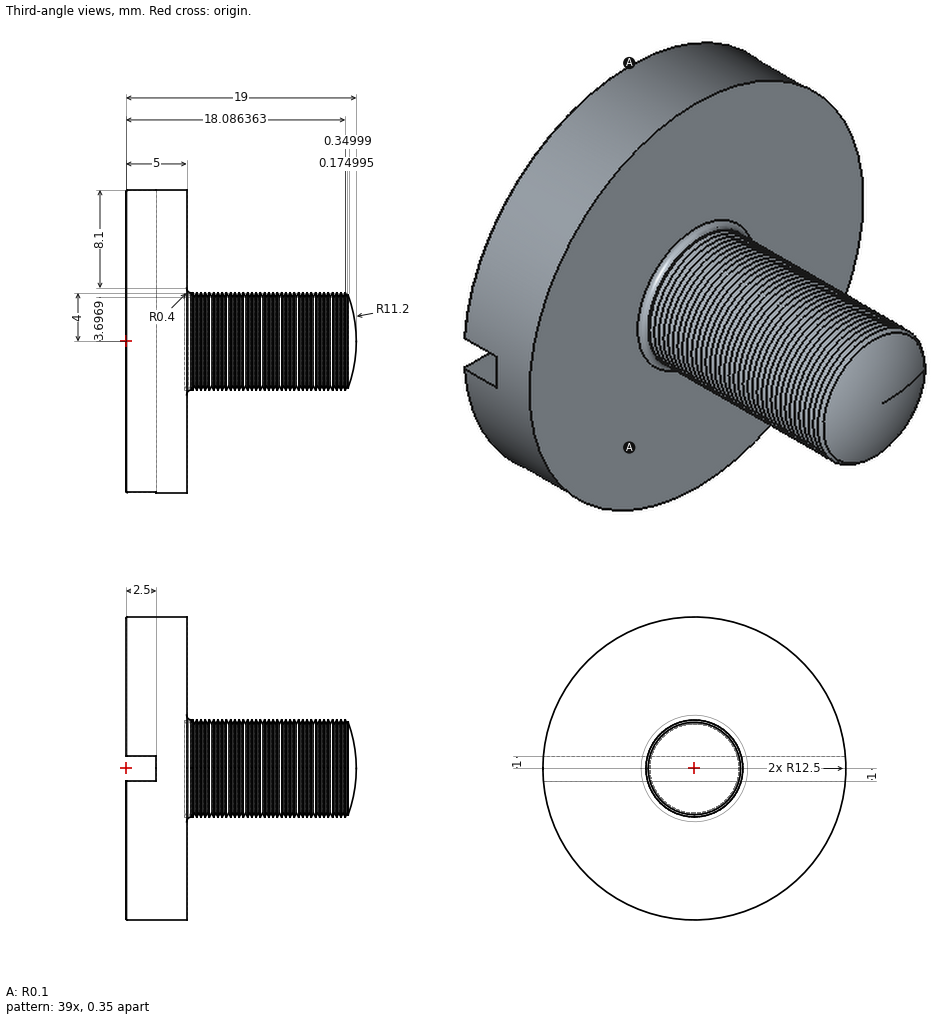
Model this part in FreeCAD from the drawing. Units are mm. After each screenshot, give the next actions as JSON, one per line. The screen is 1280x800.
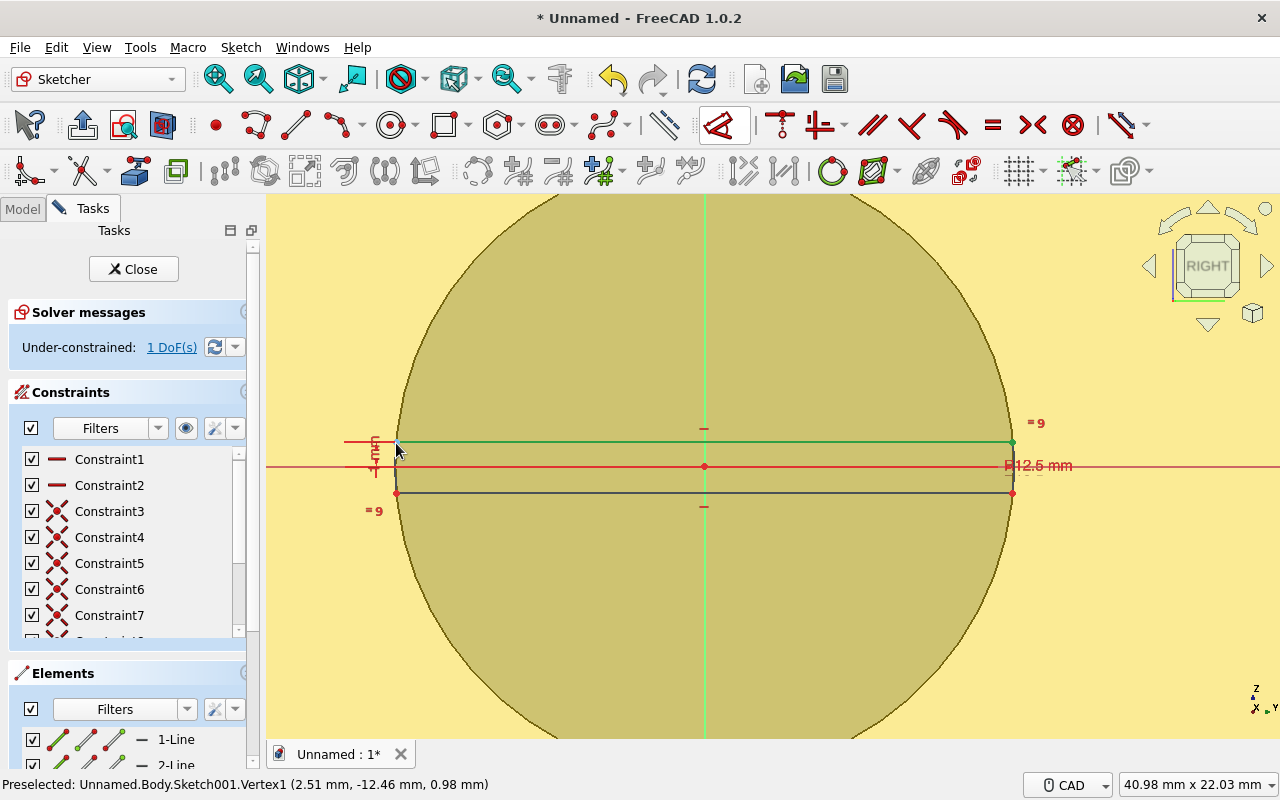
{"action": "scroll", "coordinate": [1013, 493], "scroll_direction": "up", "scroll_amount": 3}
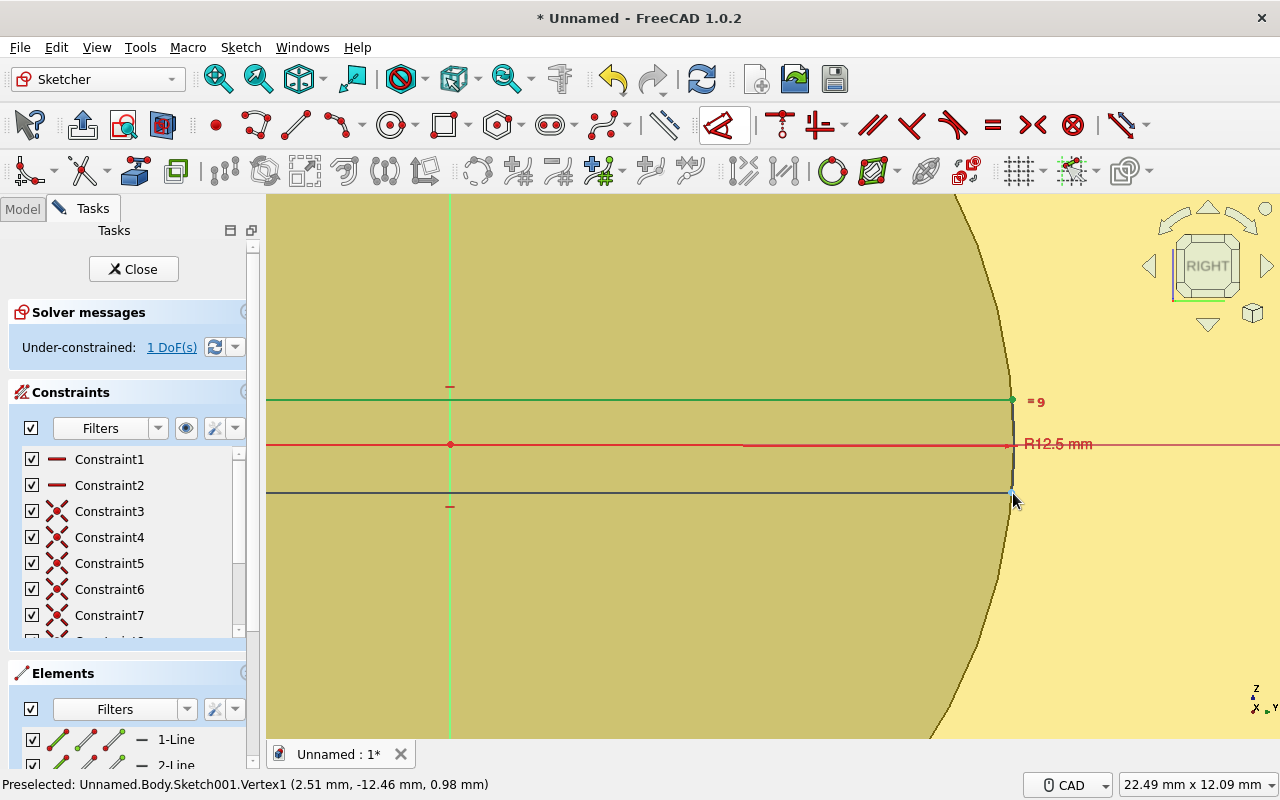
{"action": "left_click", "coordinate": [1012, 493]}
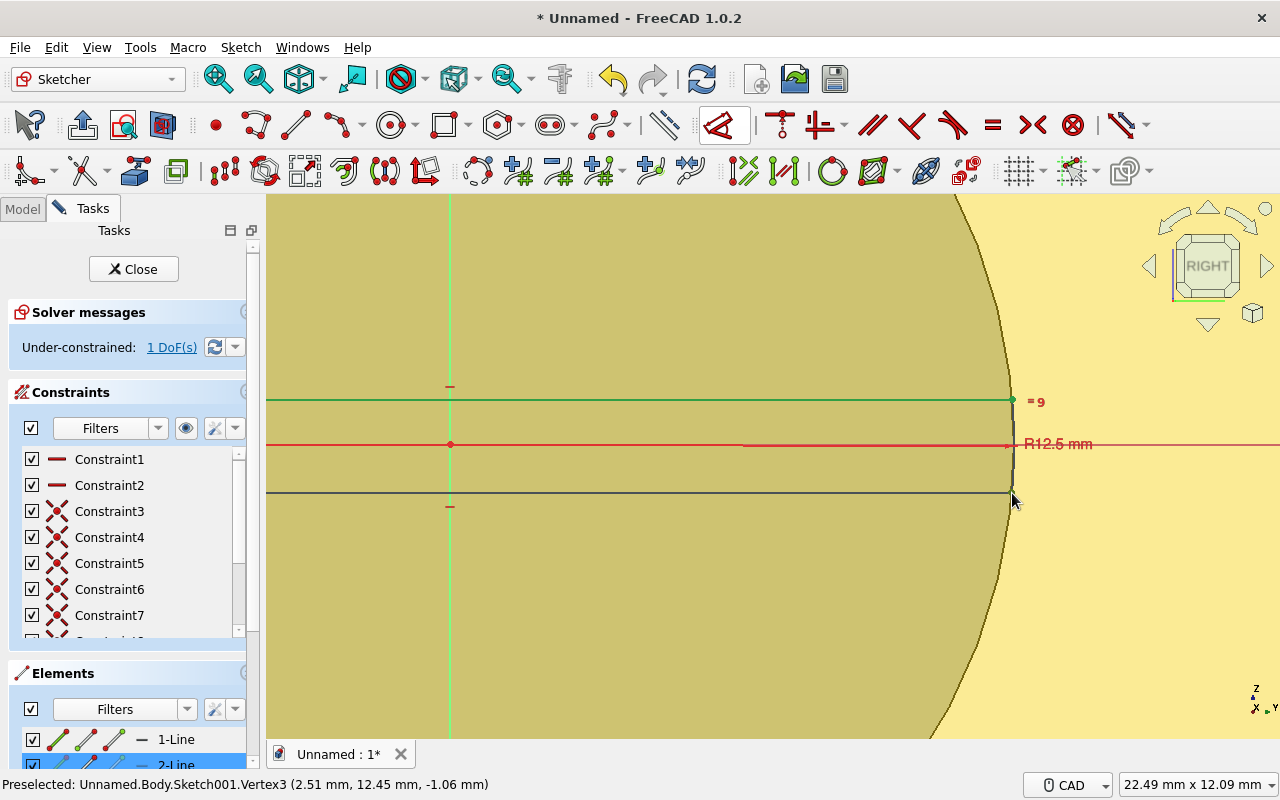
{"action": "left_click", "coordinate": [744, 126]}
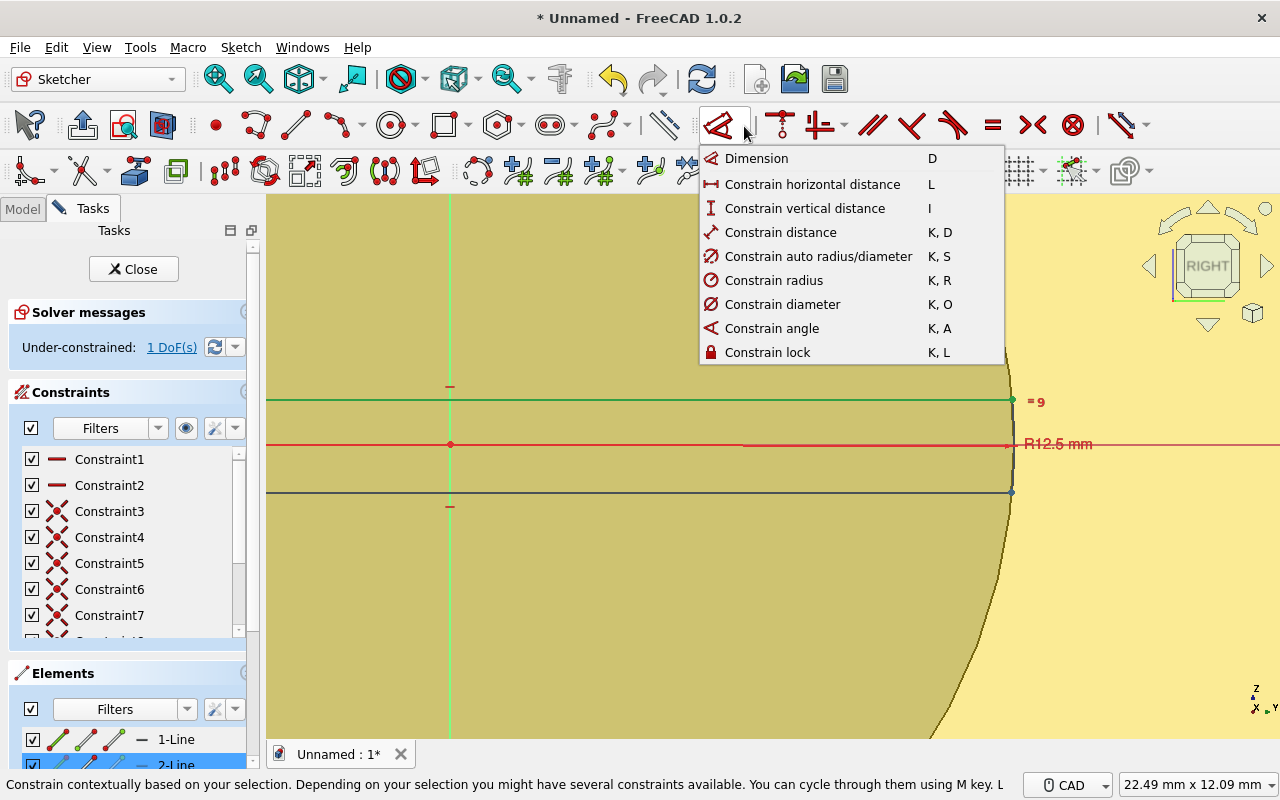
{"action": "left_click", "coordinate": [852, 208]}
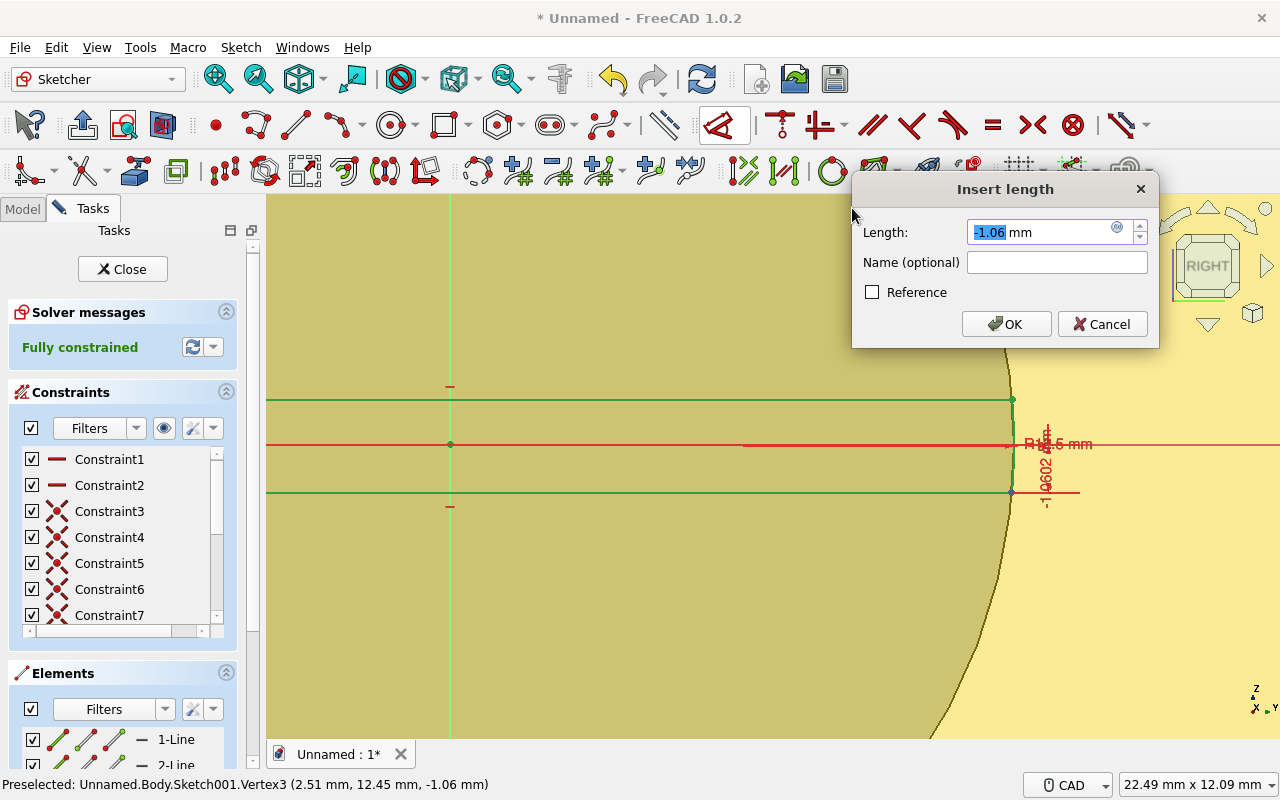
{"action": "type", "text": "-1"}
{"action": "key", "text": "Return"}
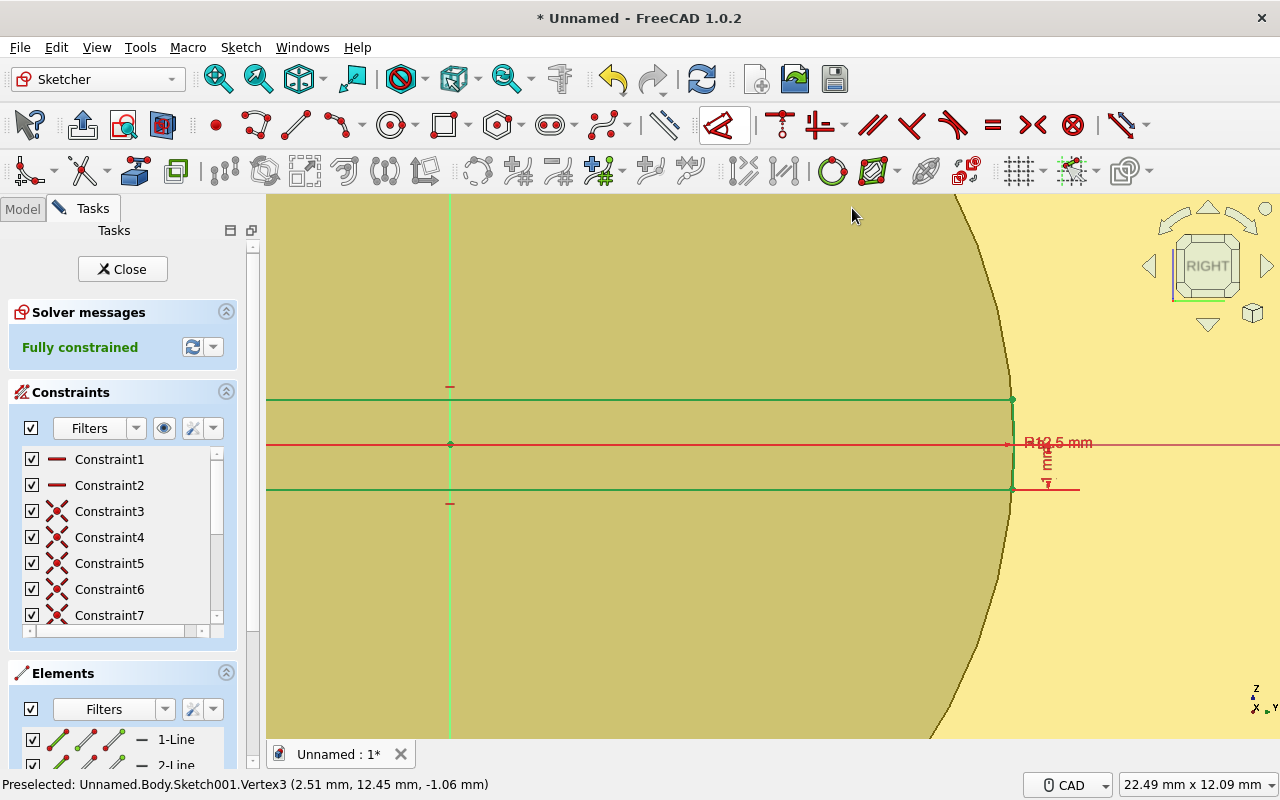
{"action": "left_click", "coordinate": [123, 269]}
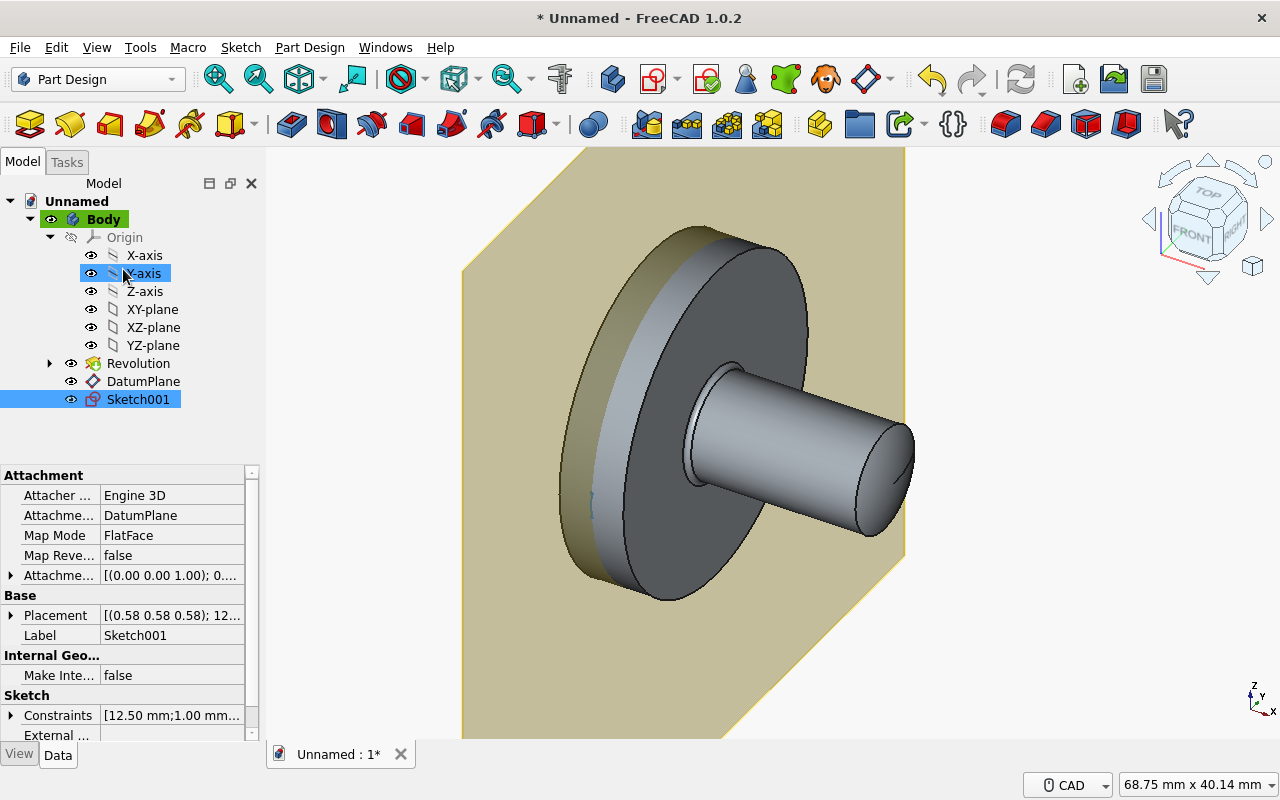
{"action": "left_click", "coordinate": [292, 124]}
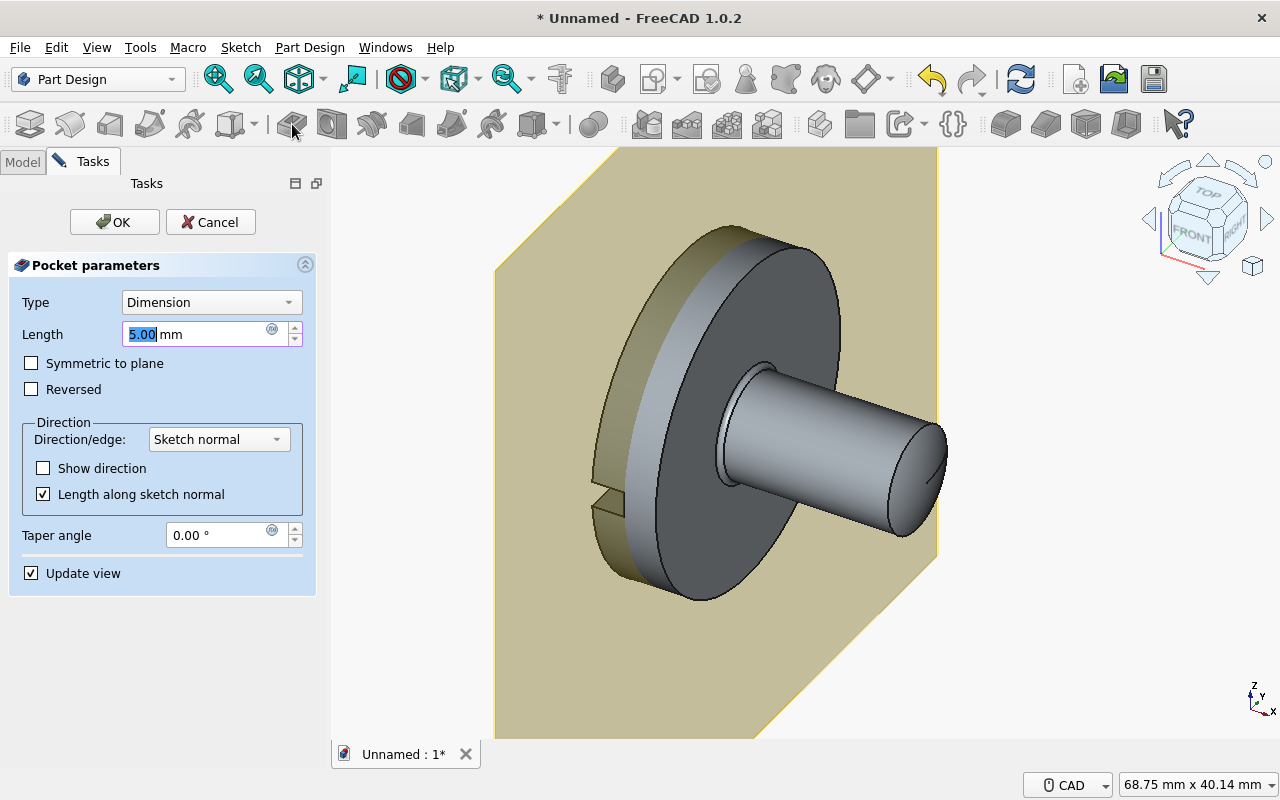
{"action": "type", "text": "2.5"}
{"action": "key", "text": "Tab"}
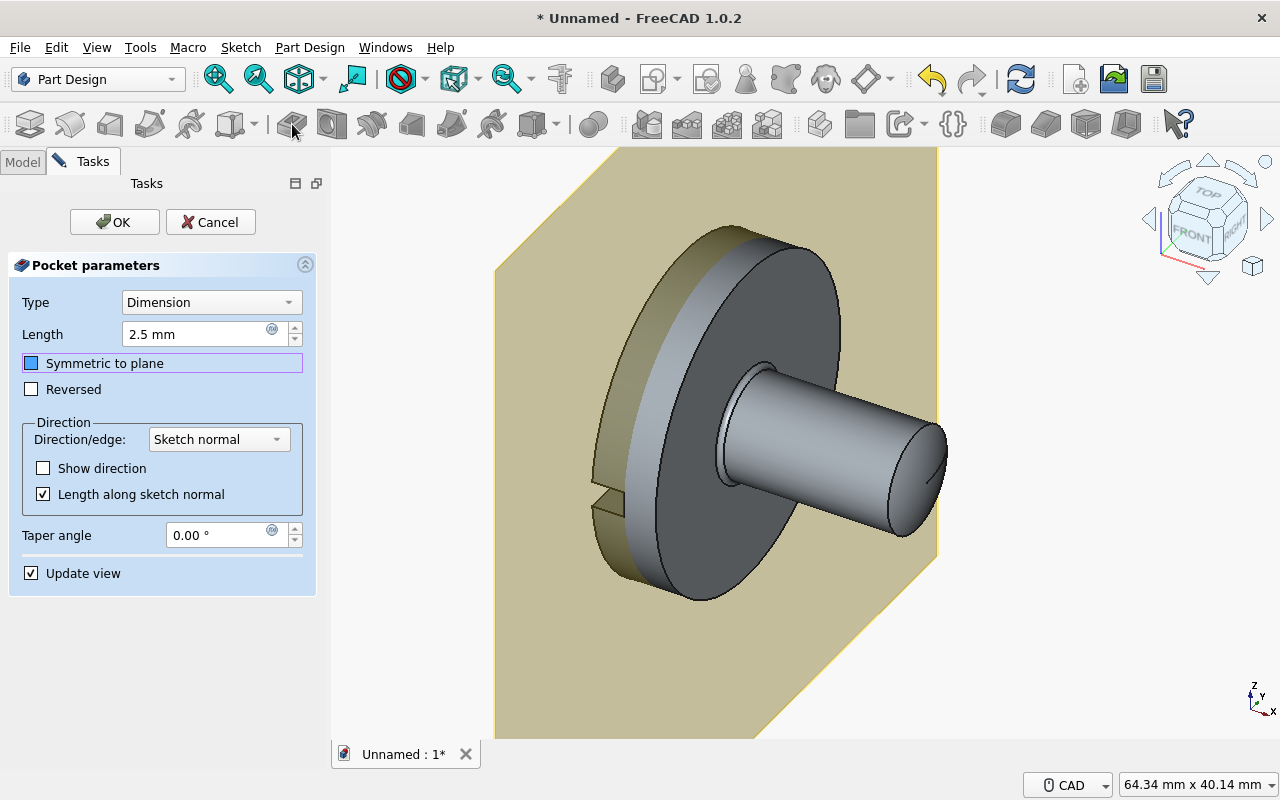
{"action": "left_click", "coordinate": [115, 222]}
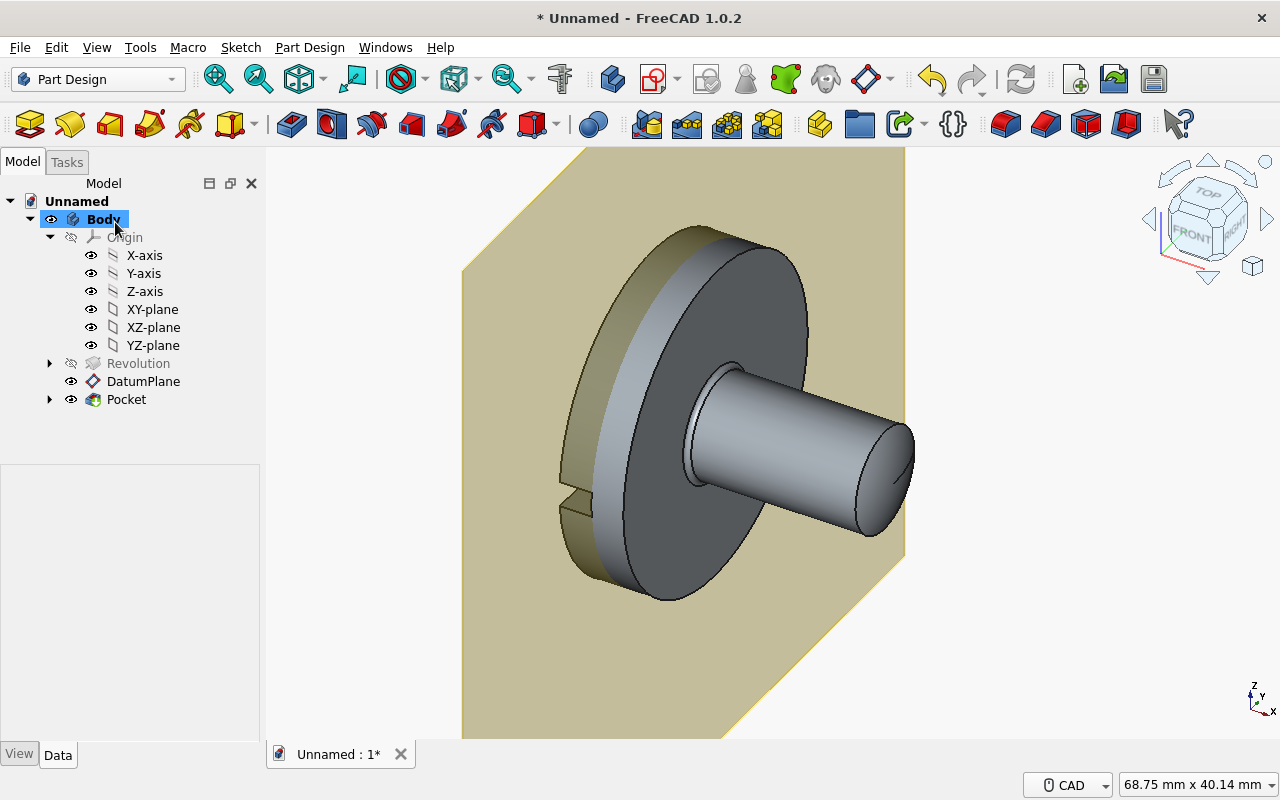
{"action": "left_click", "coordinate": [116, 381]}
{"action": "key", "text": "space"}